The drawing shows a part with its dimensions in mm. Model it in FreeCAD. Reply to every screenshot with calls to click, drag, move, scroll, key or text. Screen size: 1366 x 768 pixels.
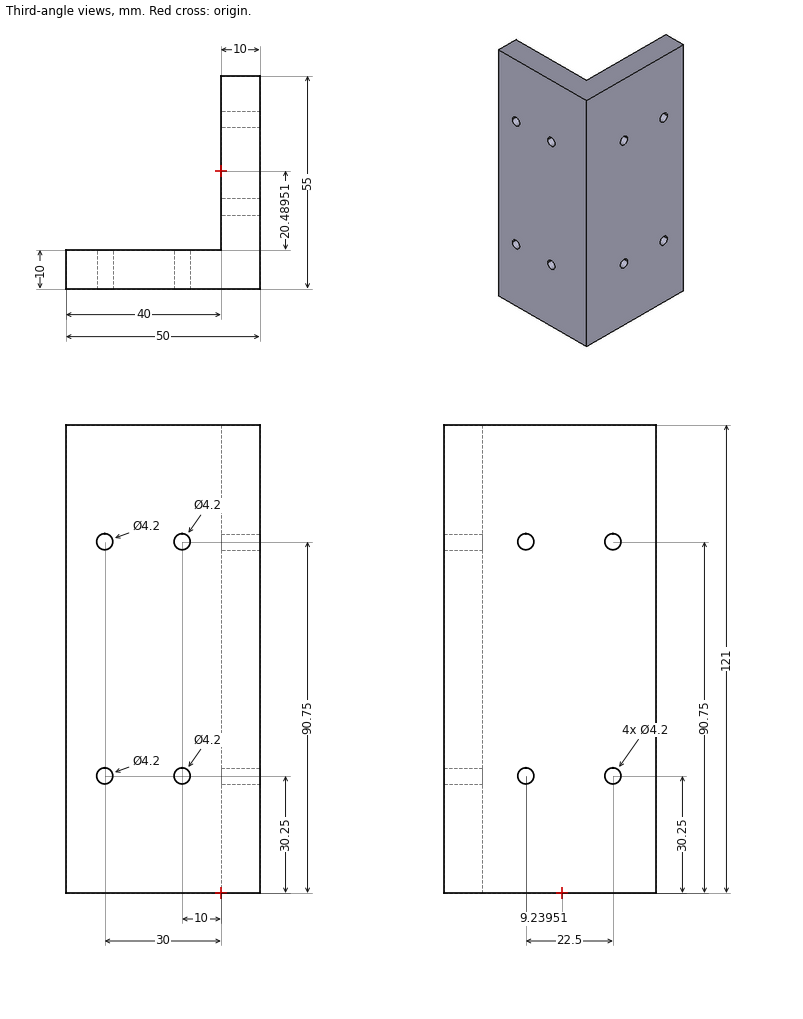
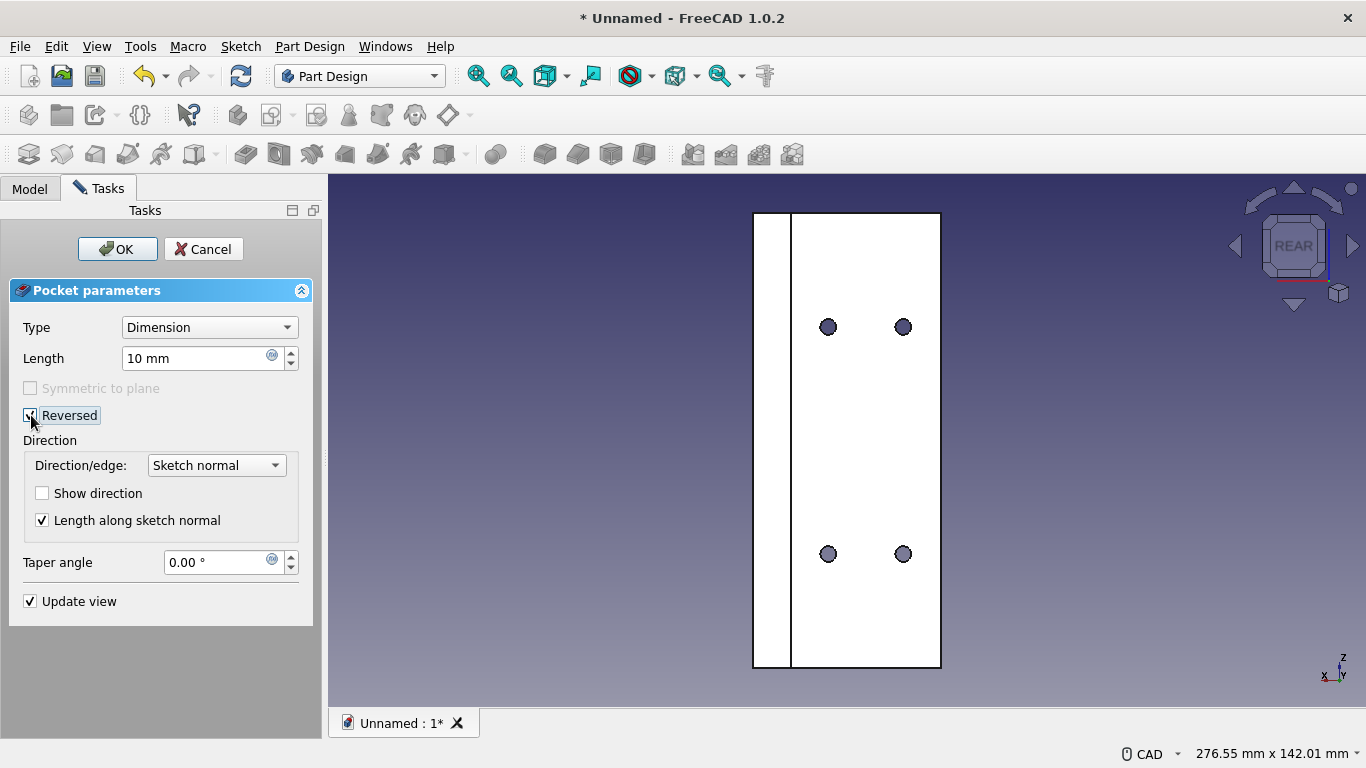
click(118, 249)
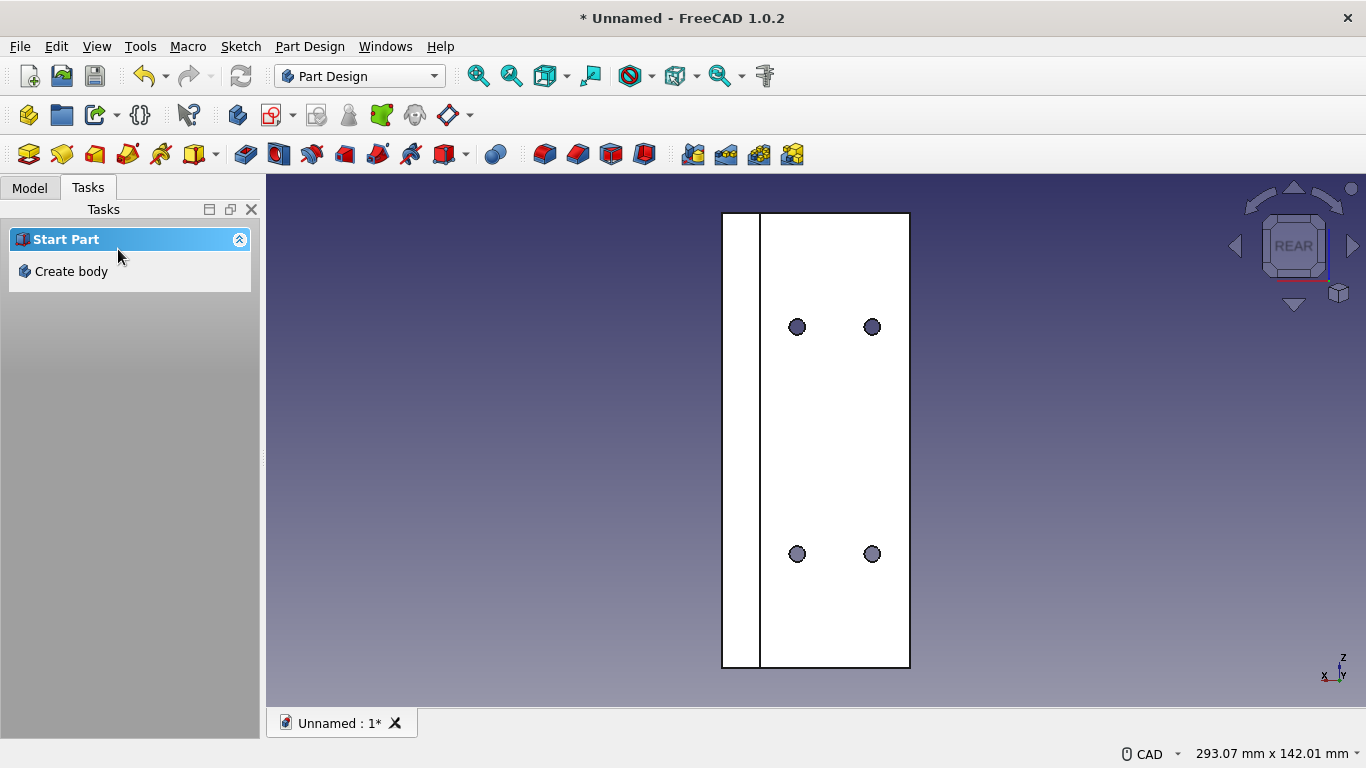
key(0)